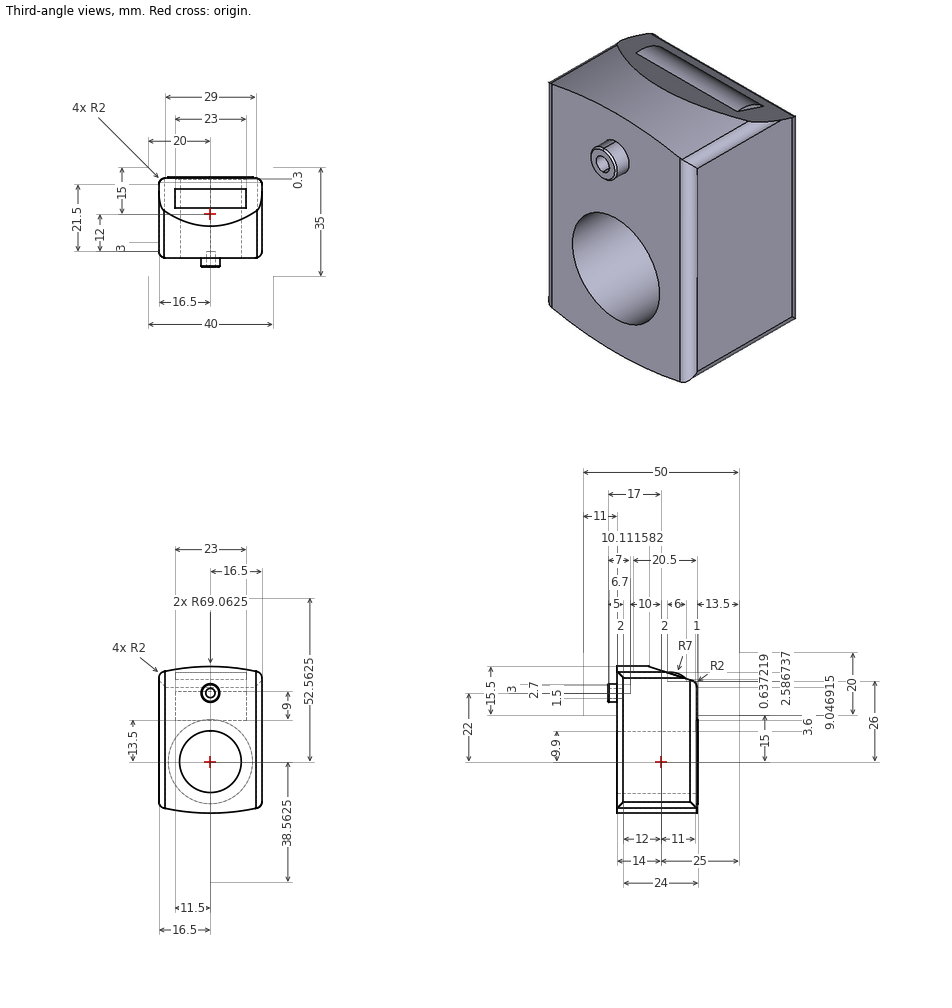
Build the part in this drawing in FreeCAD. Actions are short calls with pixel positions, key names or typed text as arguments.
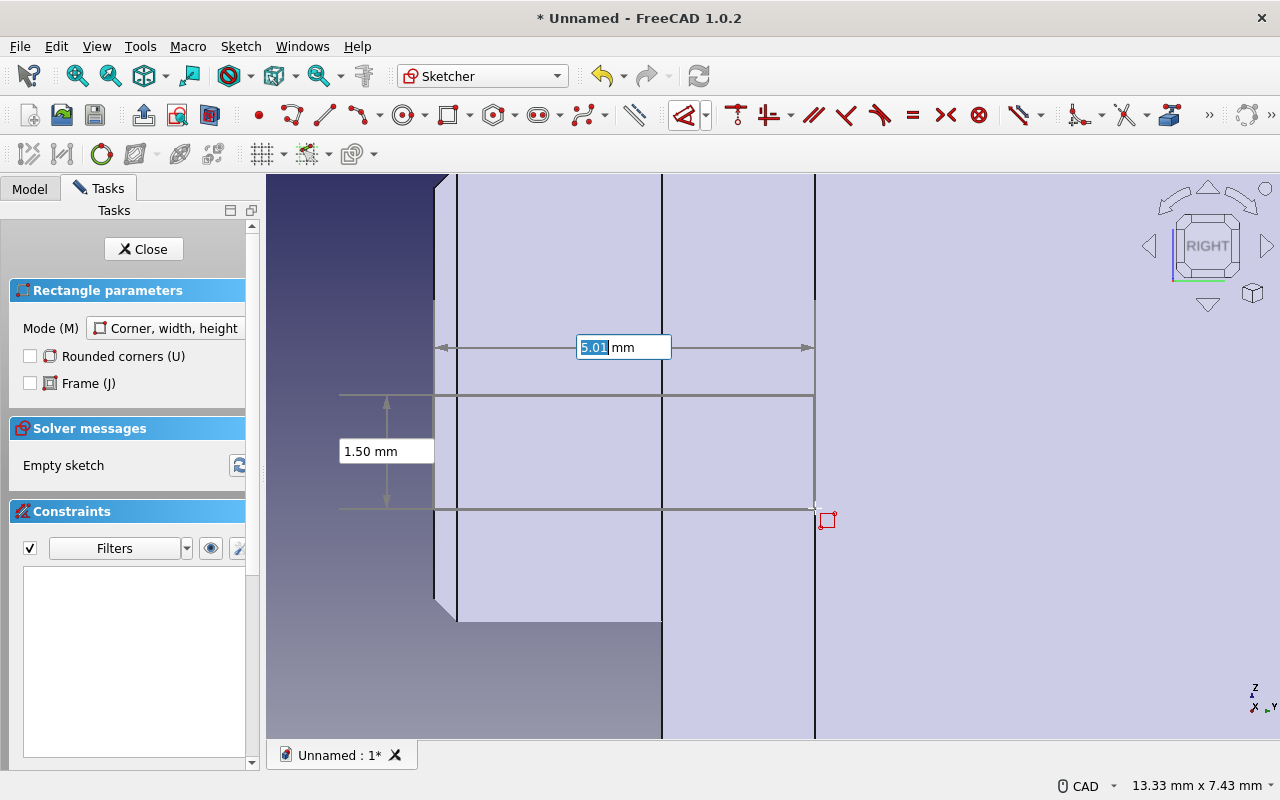
text(5)
key(Tab)
text(1.5)
key(Return)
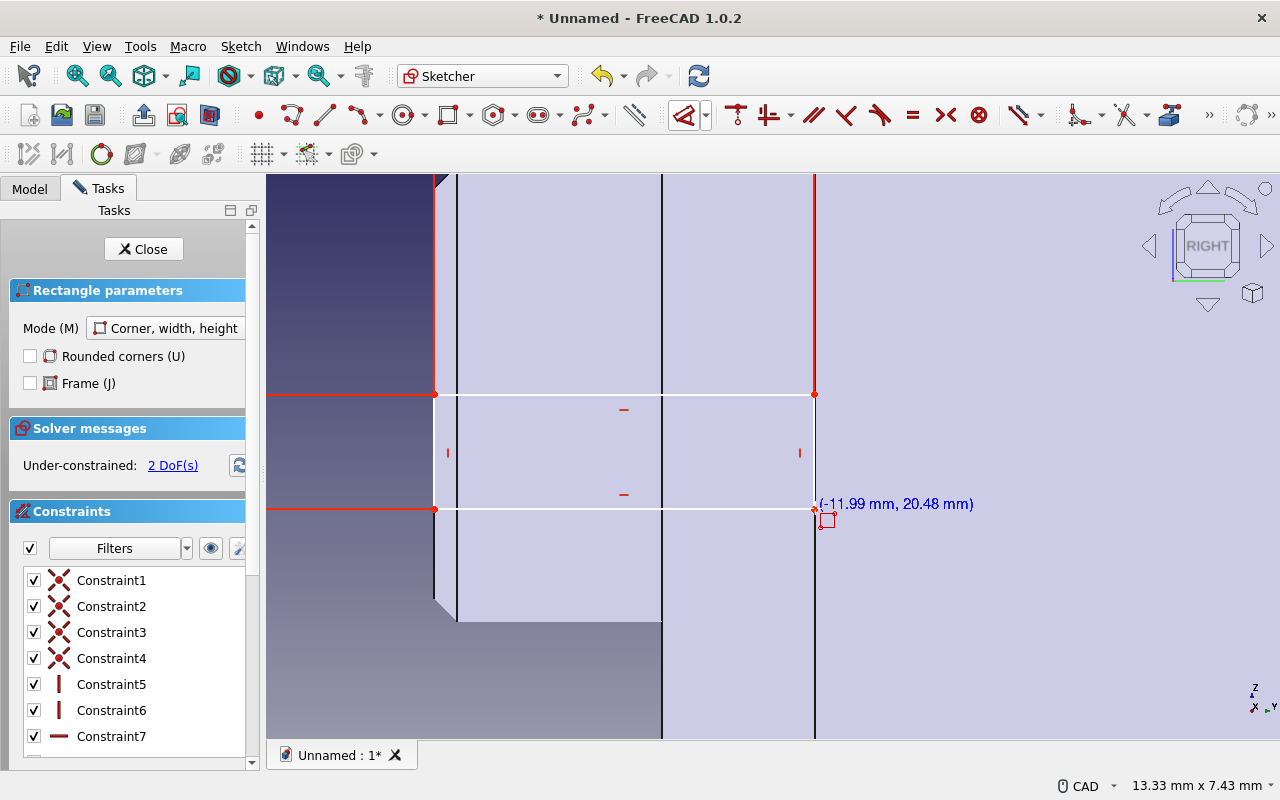
click(325, 116)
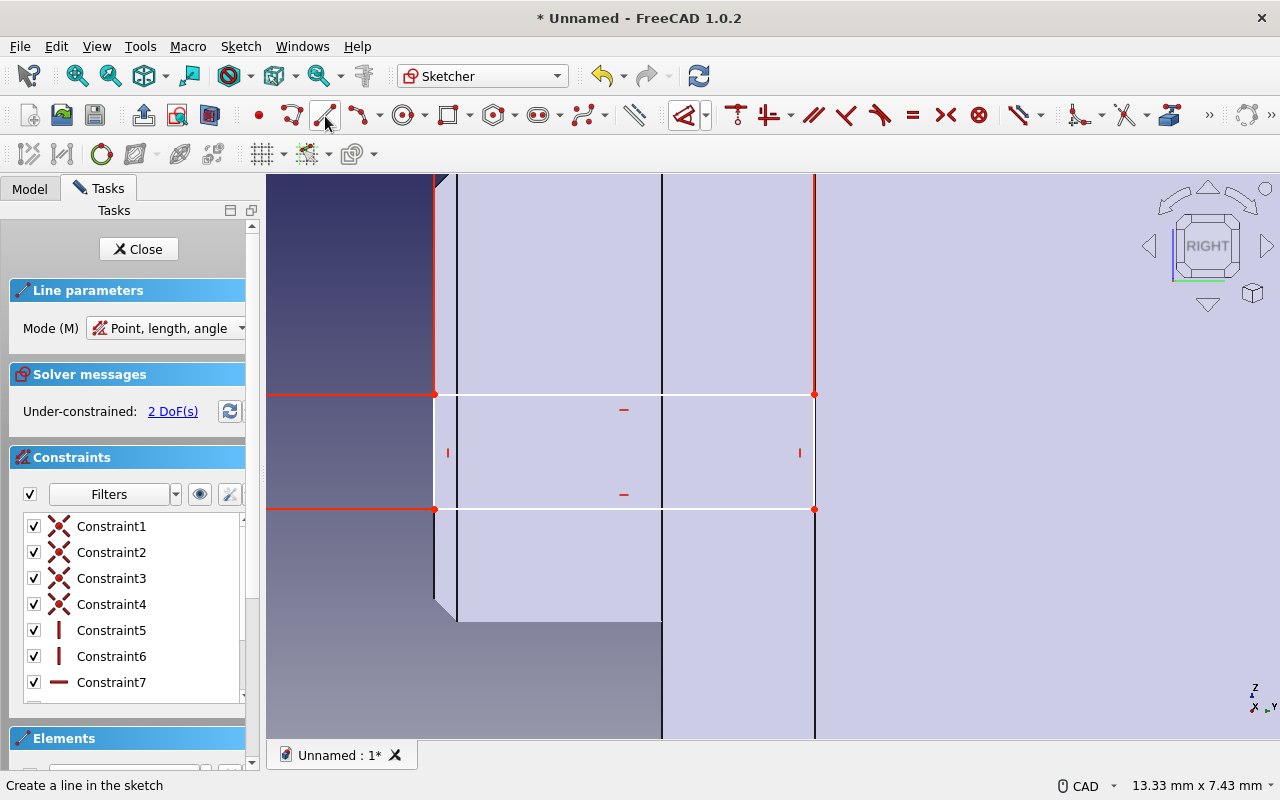
click(853, 394)
click(967, 394)
key(Escape)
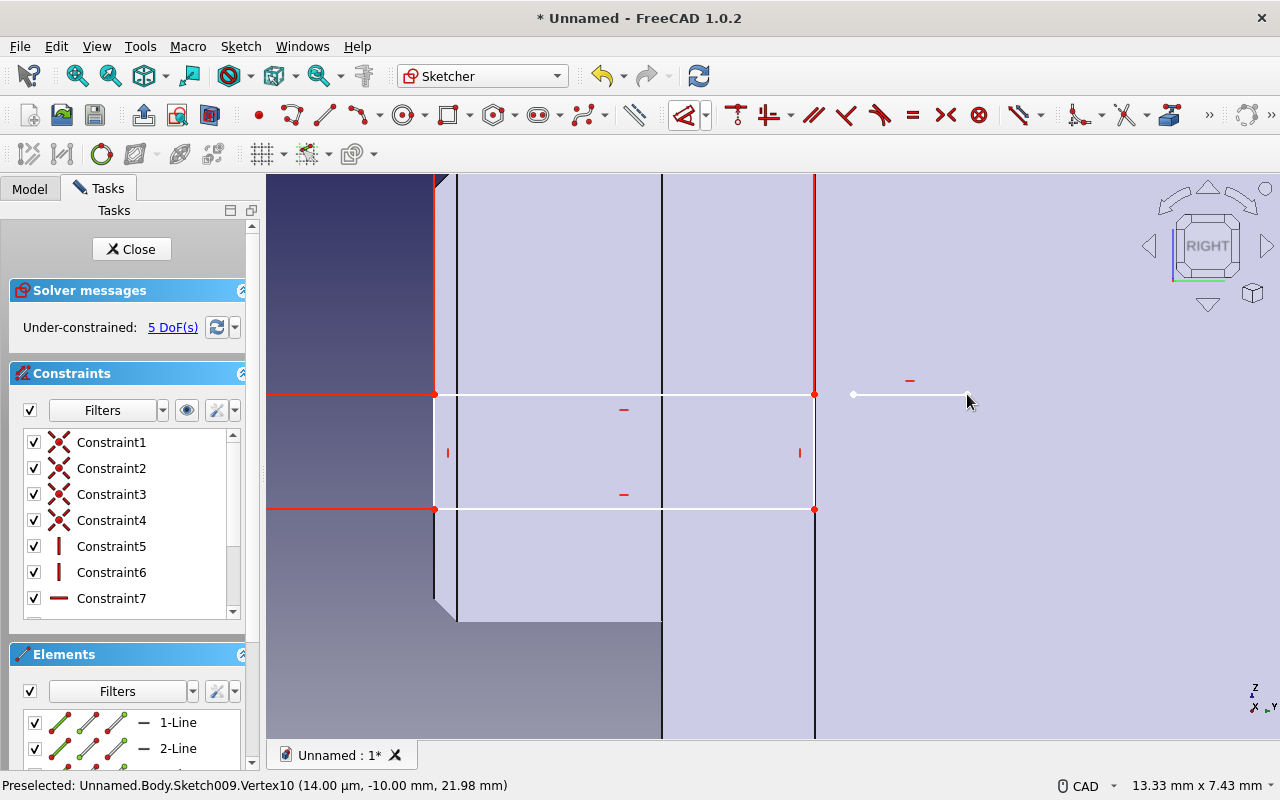
click(887, 395)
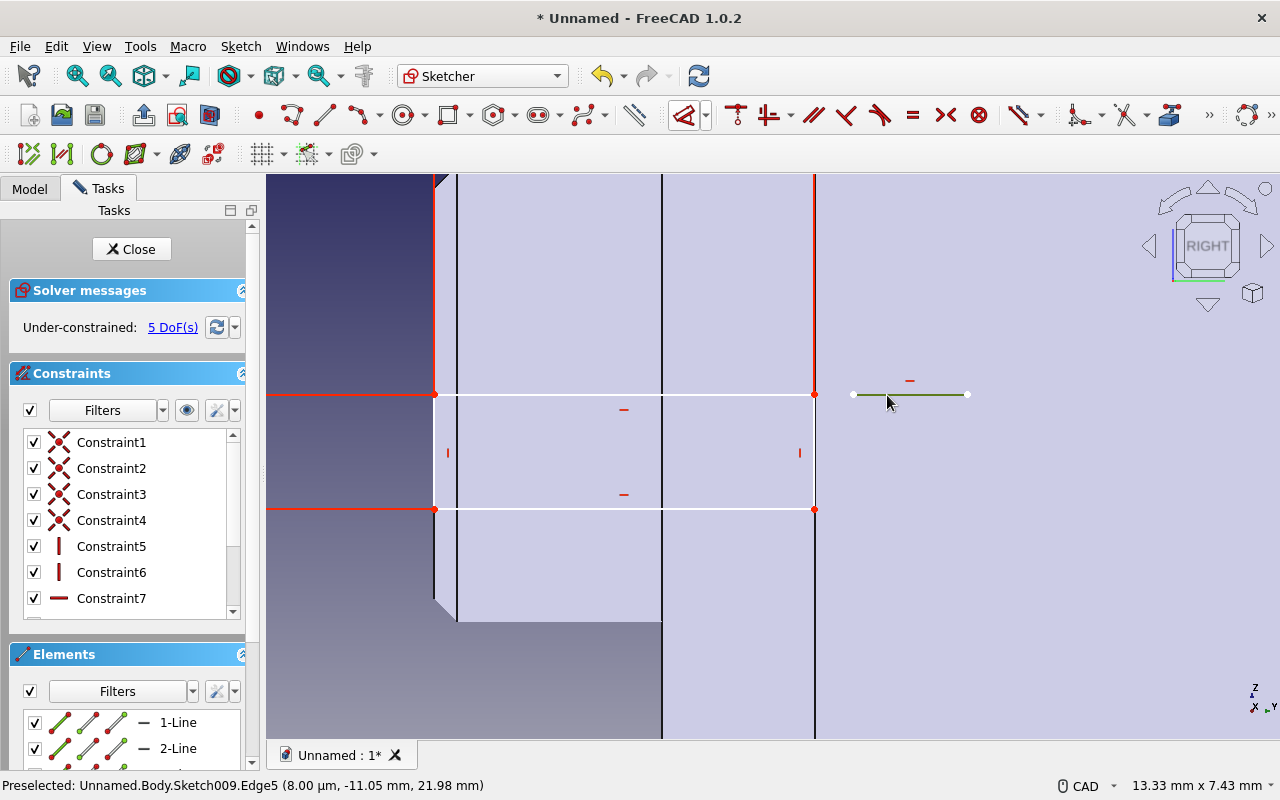
click(635, 116)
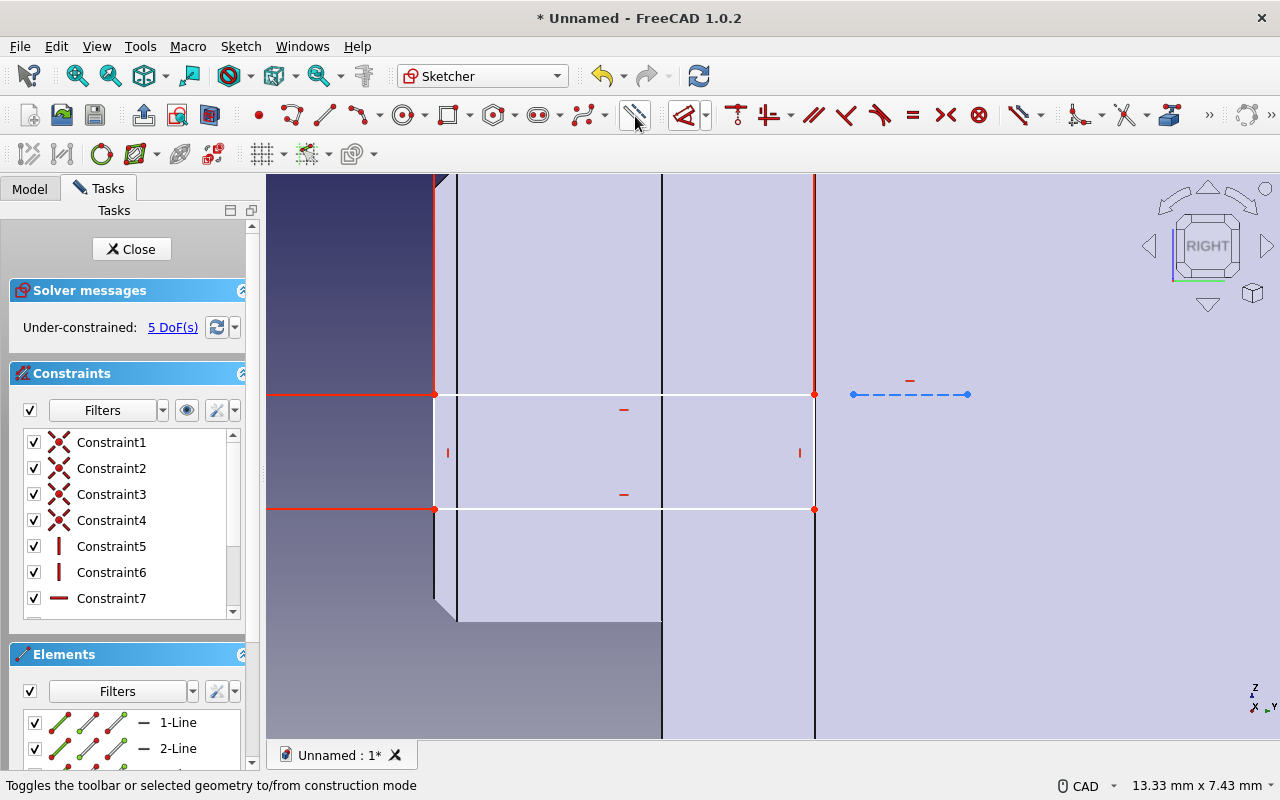
click(434, 395)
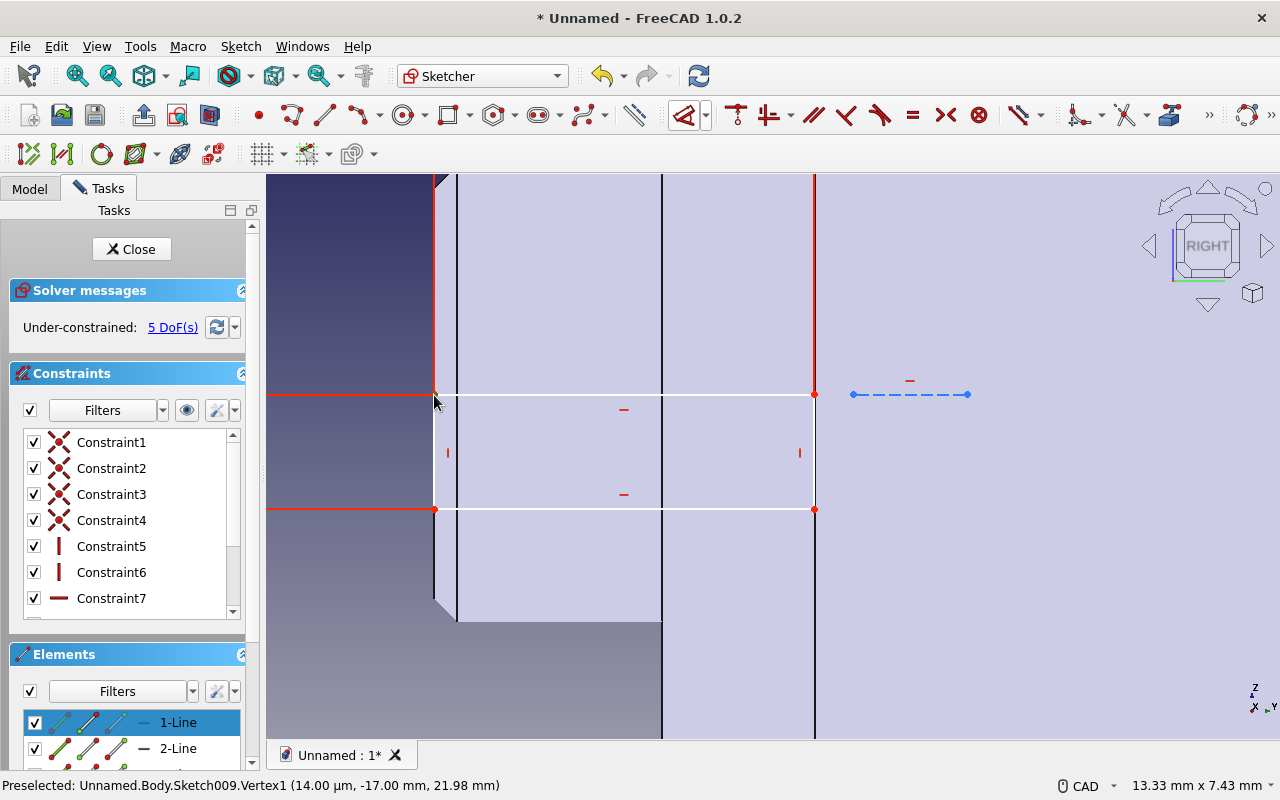
click(706, 116)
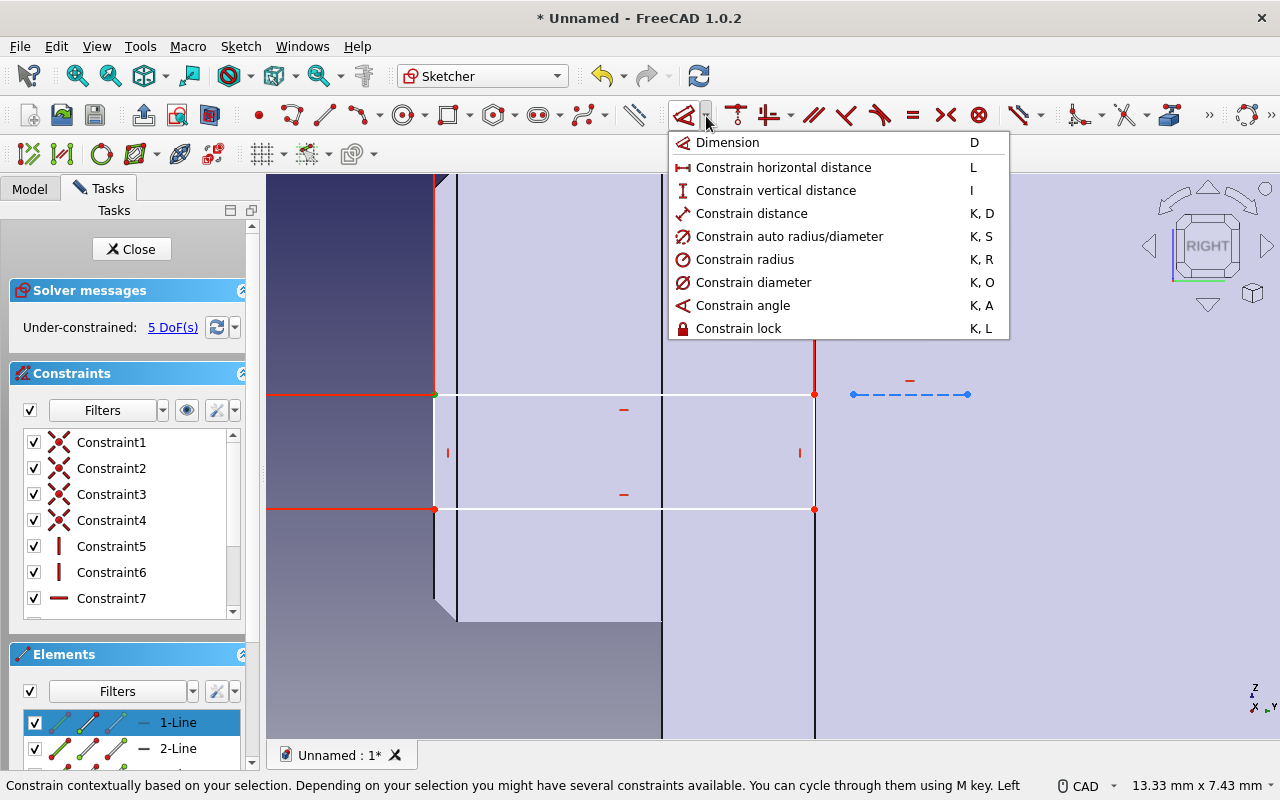
click(839, 168)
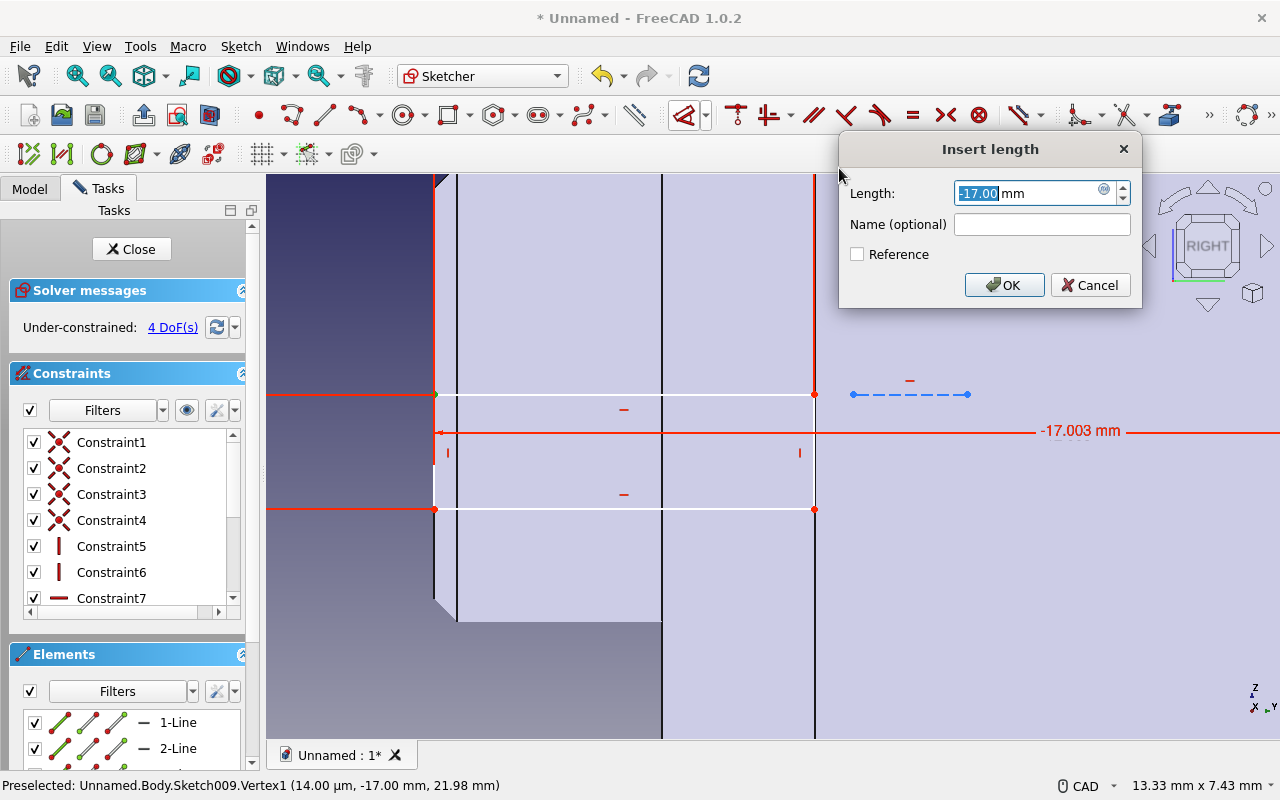
text(-17)
key(Return)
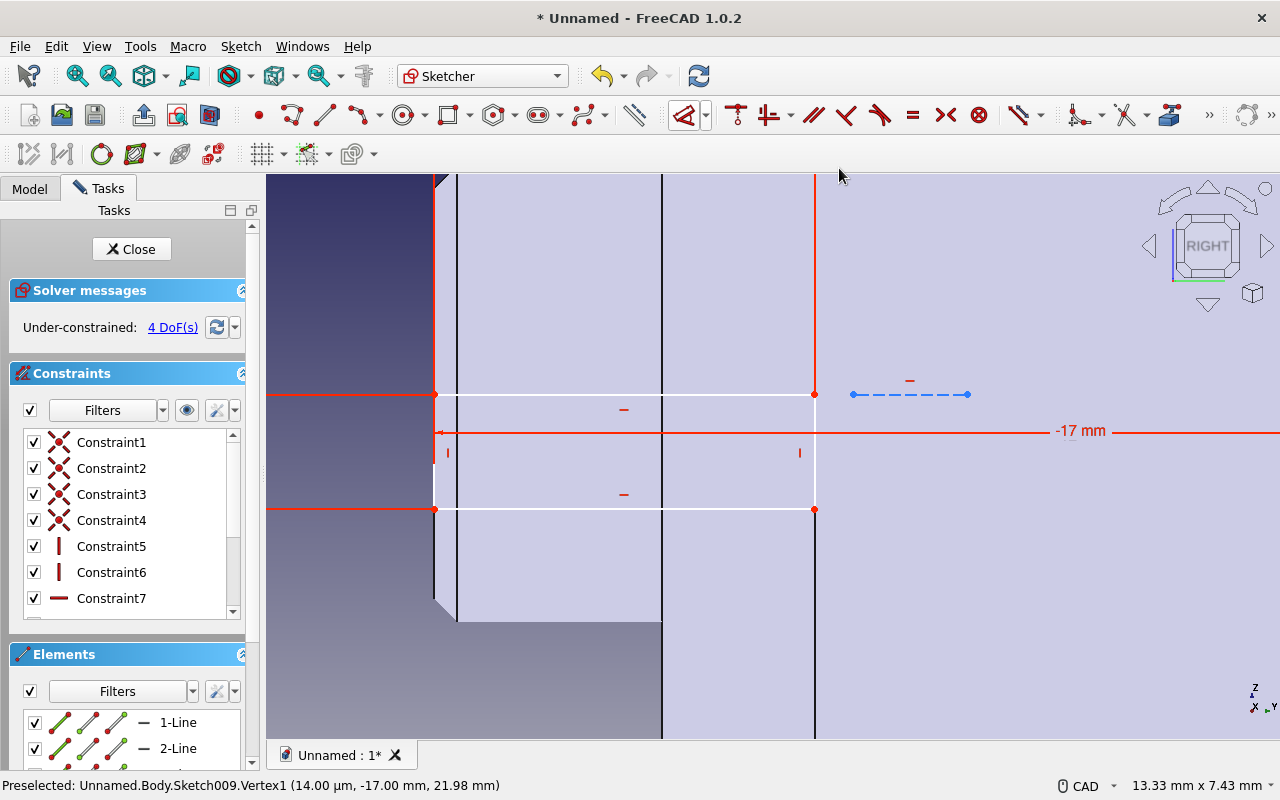
click(434, 395)